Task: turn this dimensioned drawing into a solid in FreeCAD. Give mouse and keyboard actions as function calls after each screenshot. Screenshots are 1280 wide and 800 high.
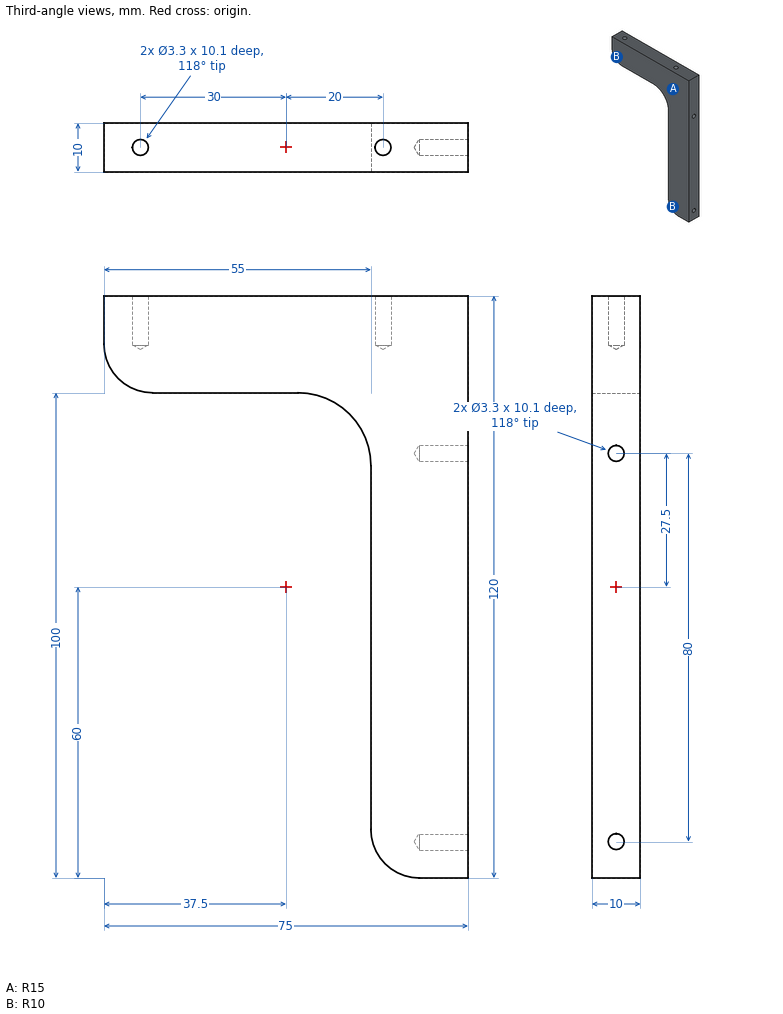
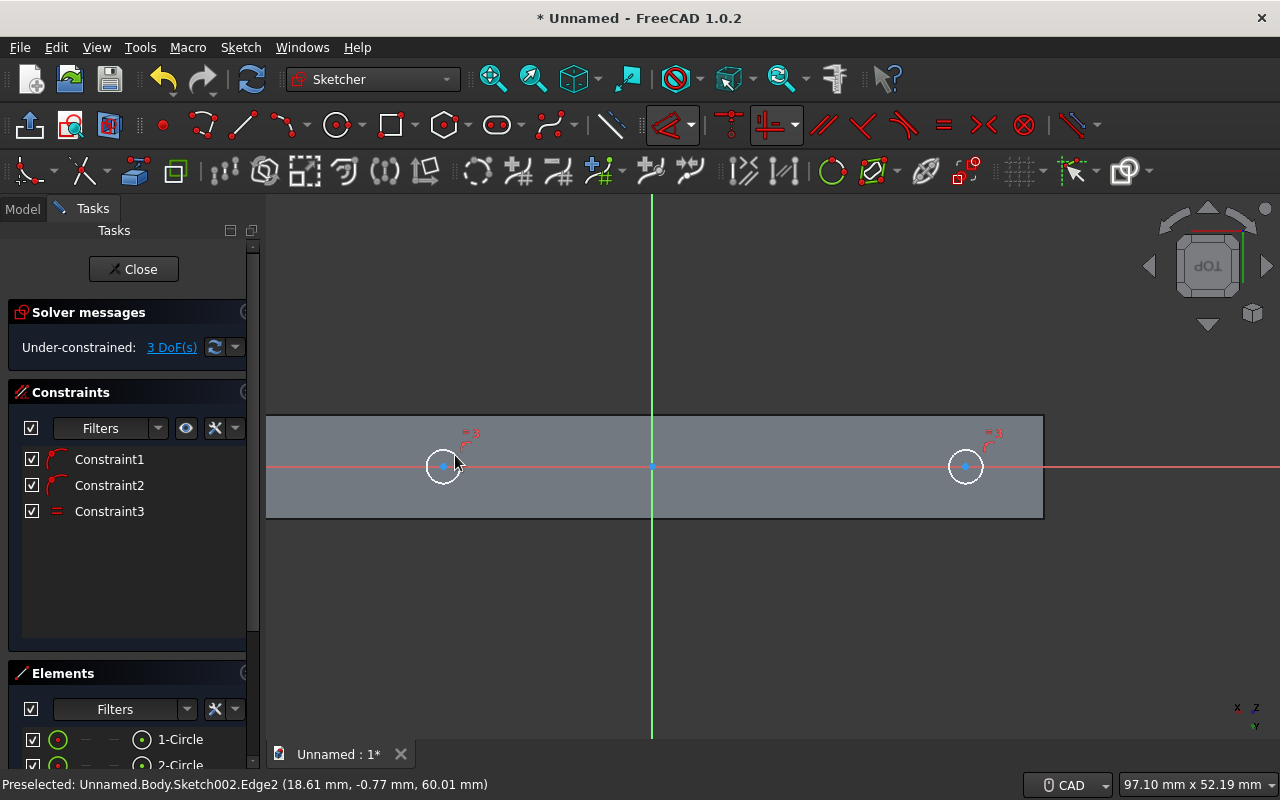
key(d)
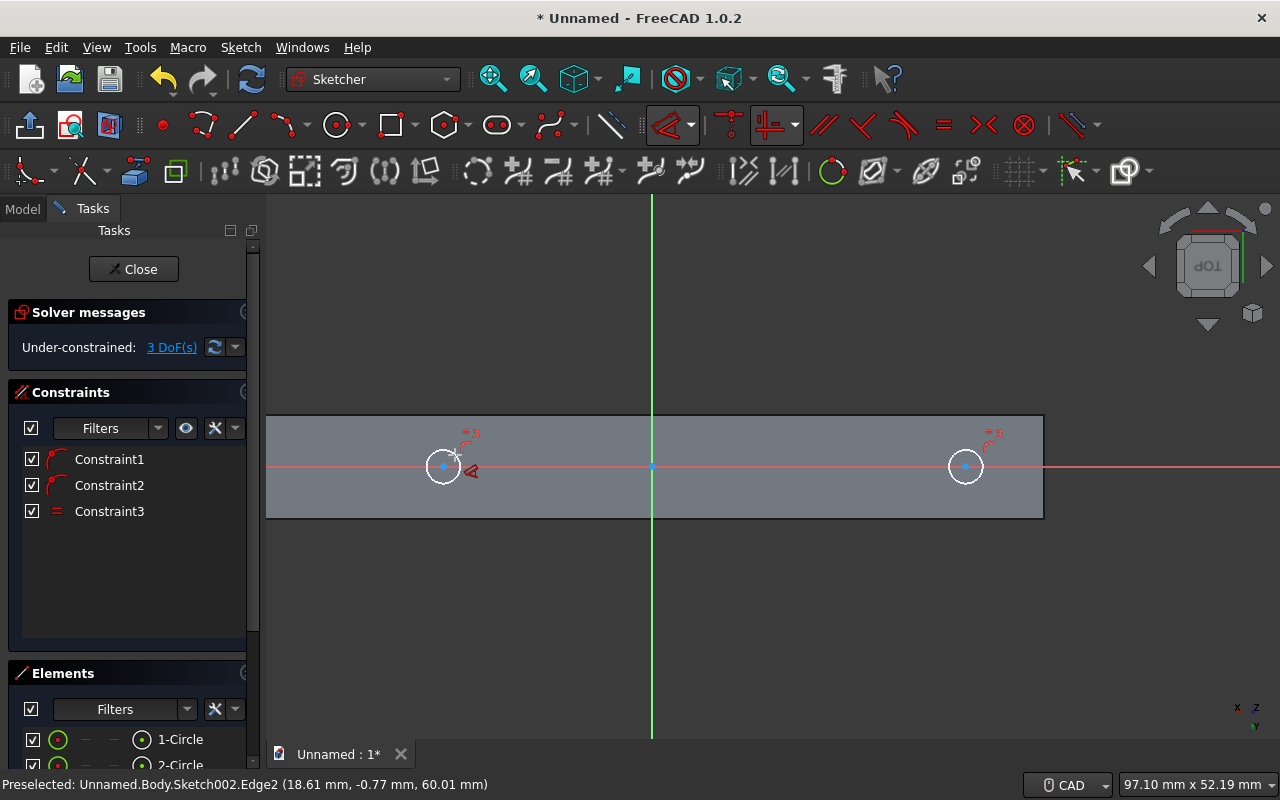
click(978, 455)
click(1001, 433)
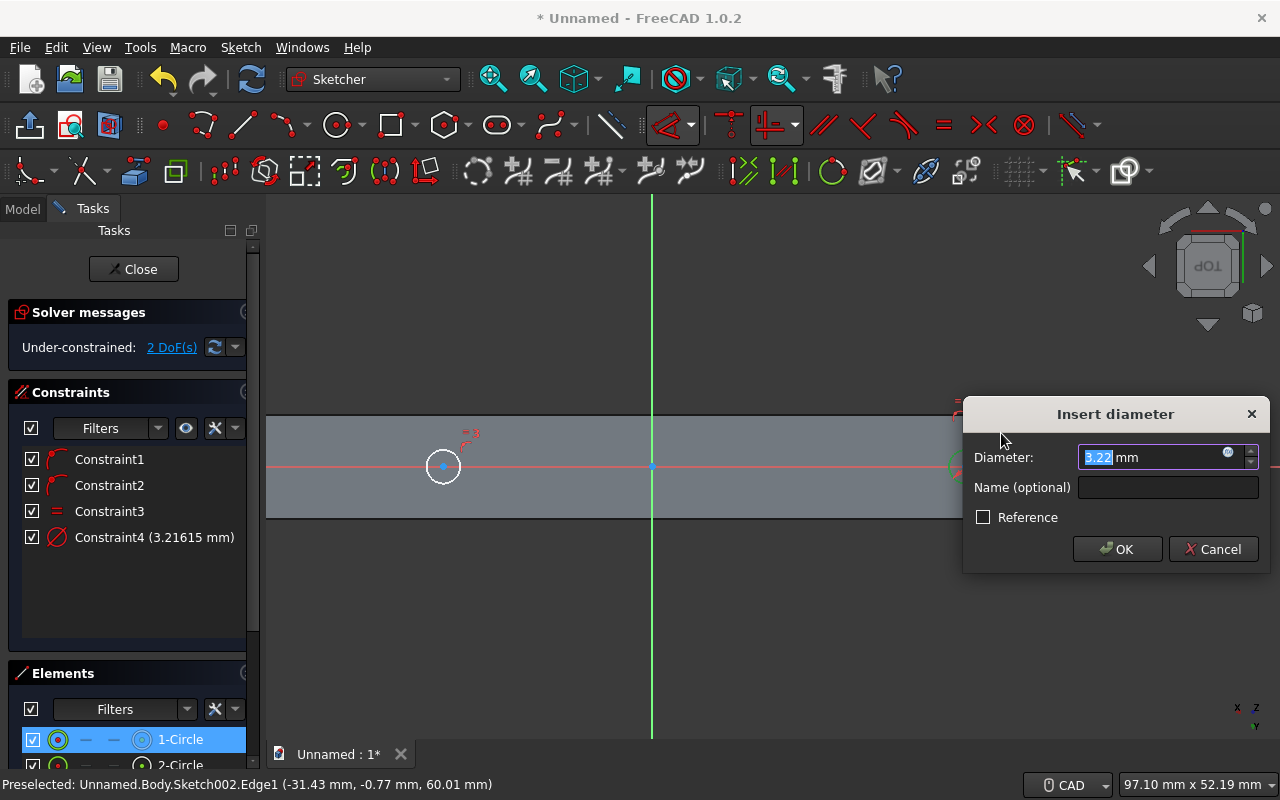
text(3.3)
key(Return)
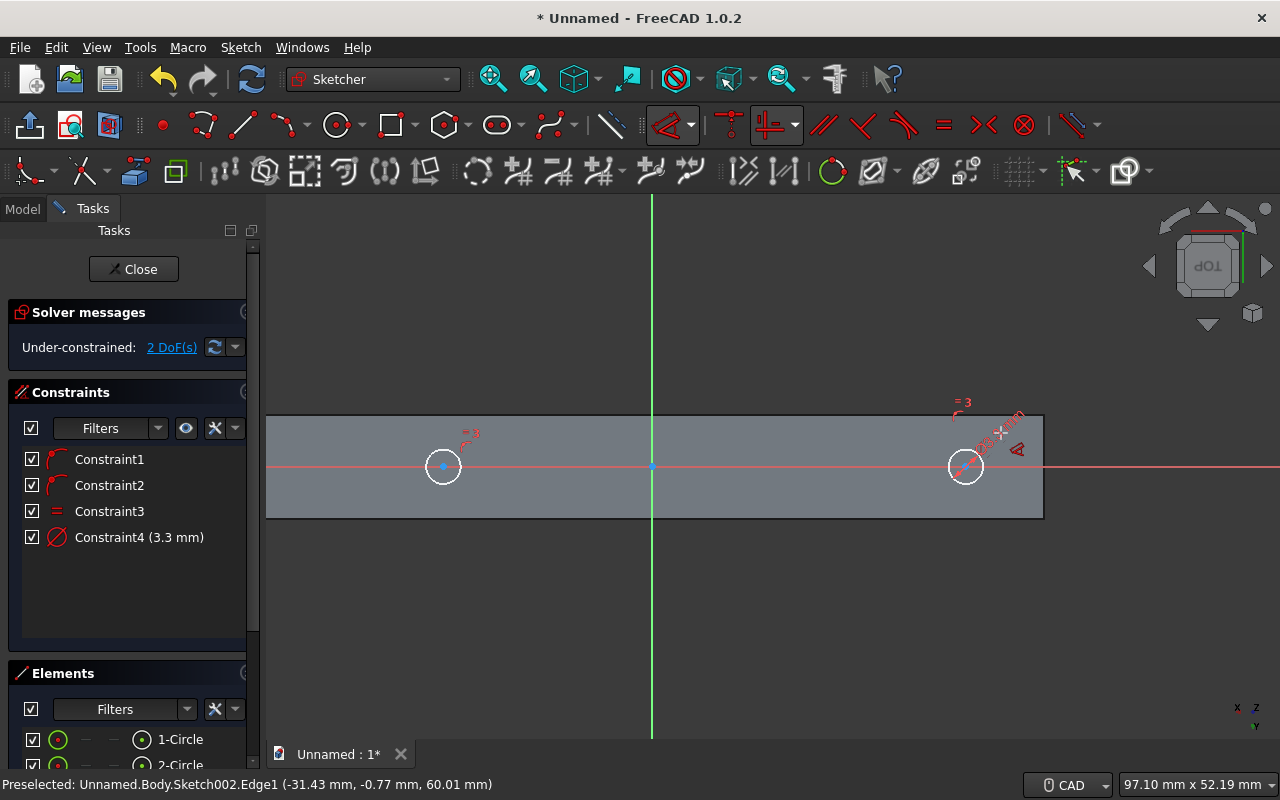
click(966, 467)
click(809, 501)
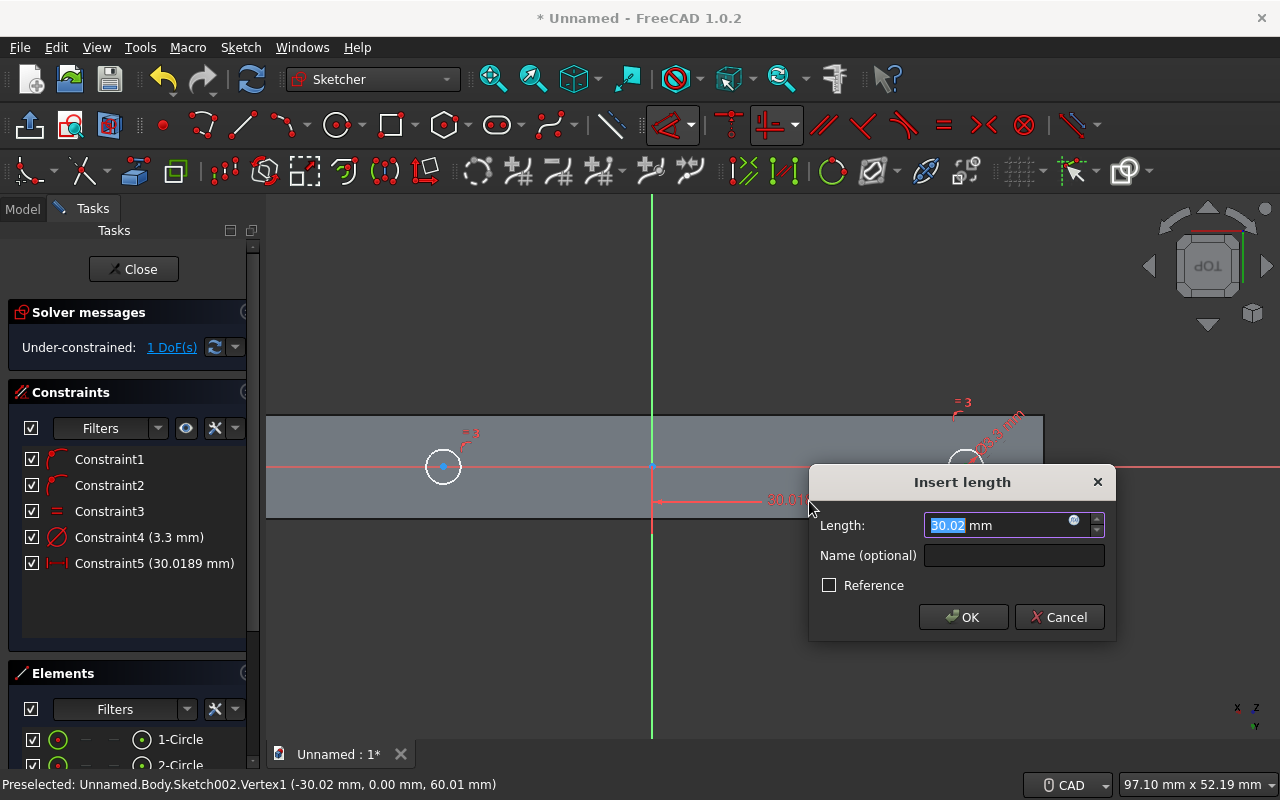
text(30)
key(Return)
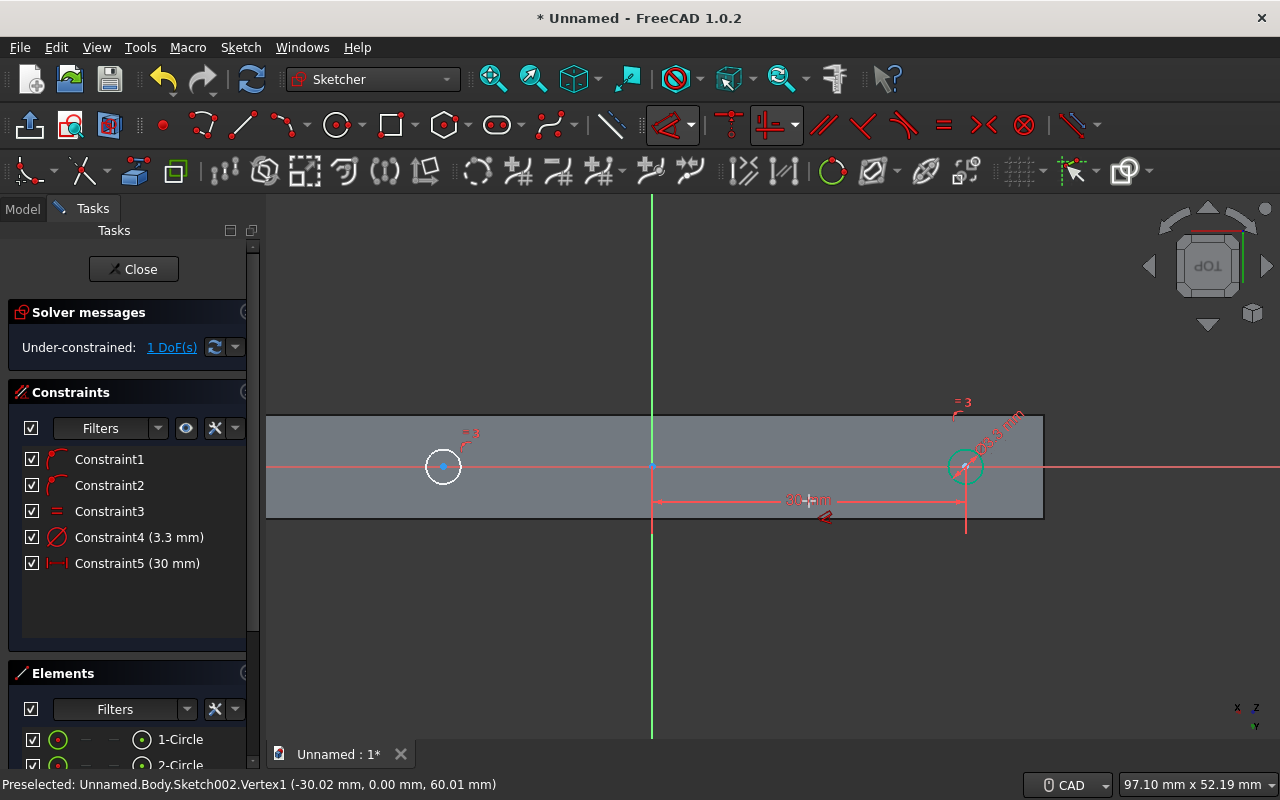
click(443, 467)
click(548, 501)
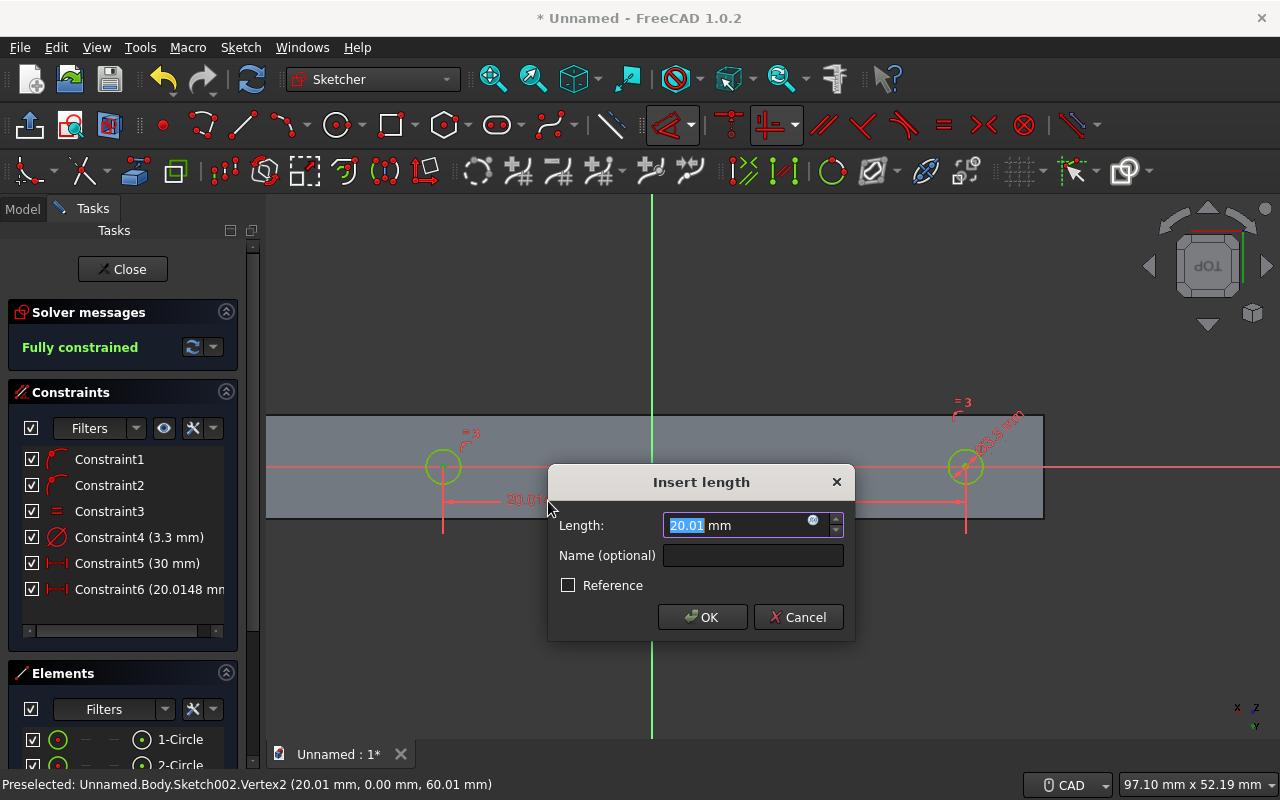
text(20)
key(Return)
key(Escape)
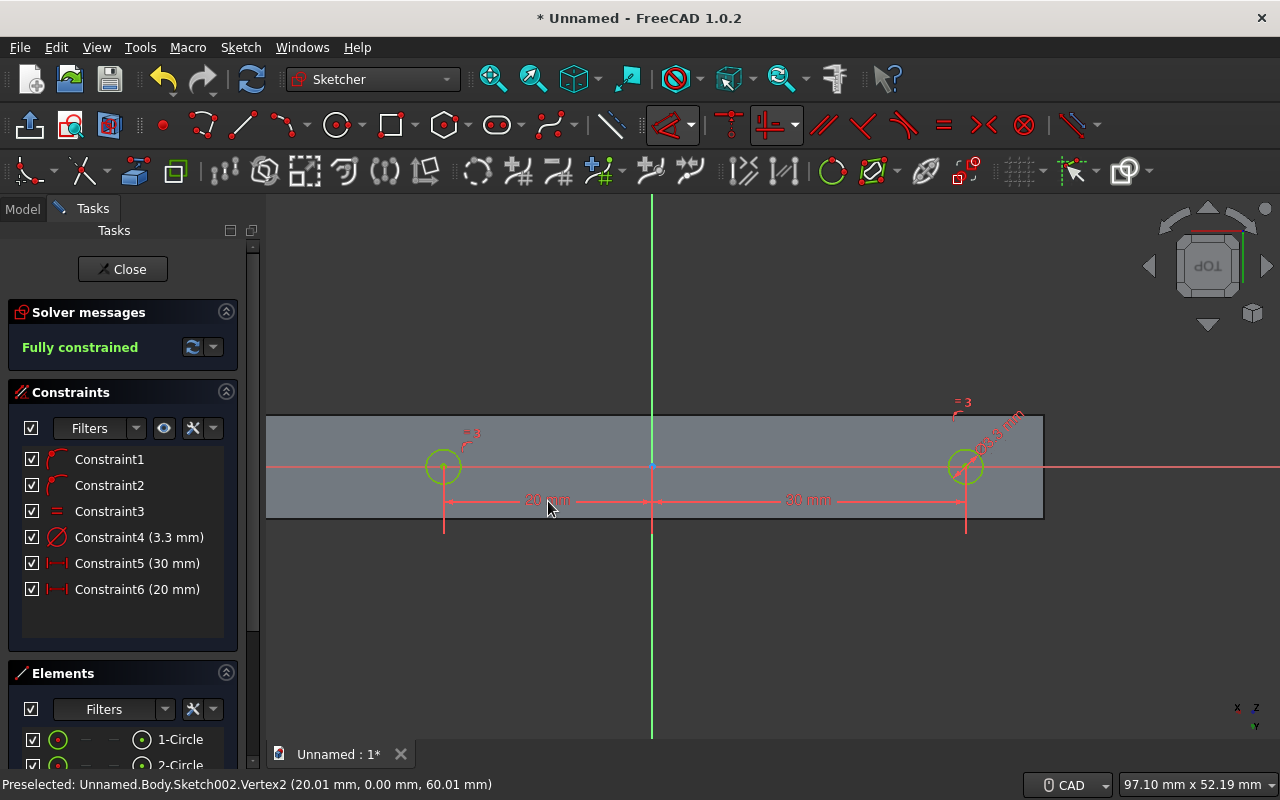
click(123, 269)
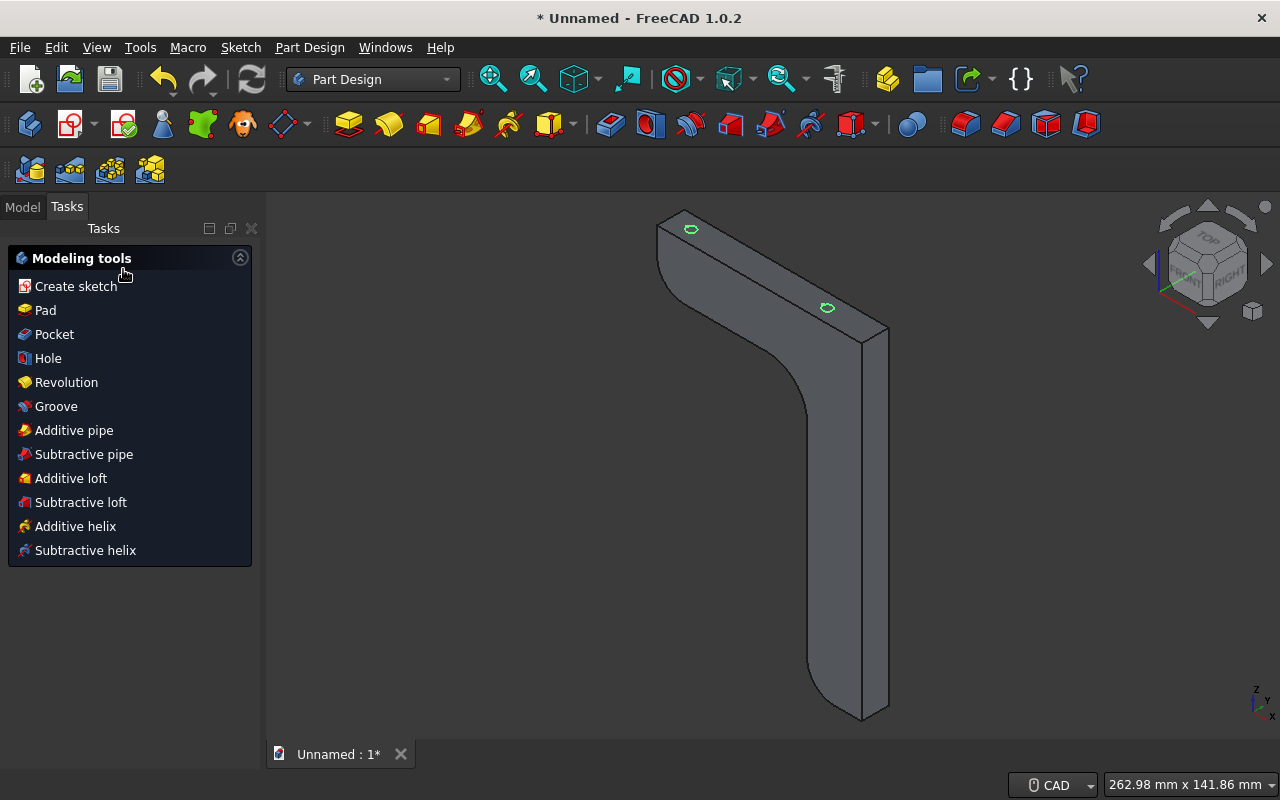
click(652, 124)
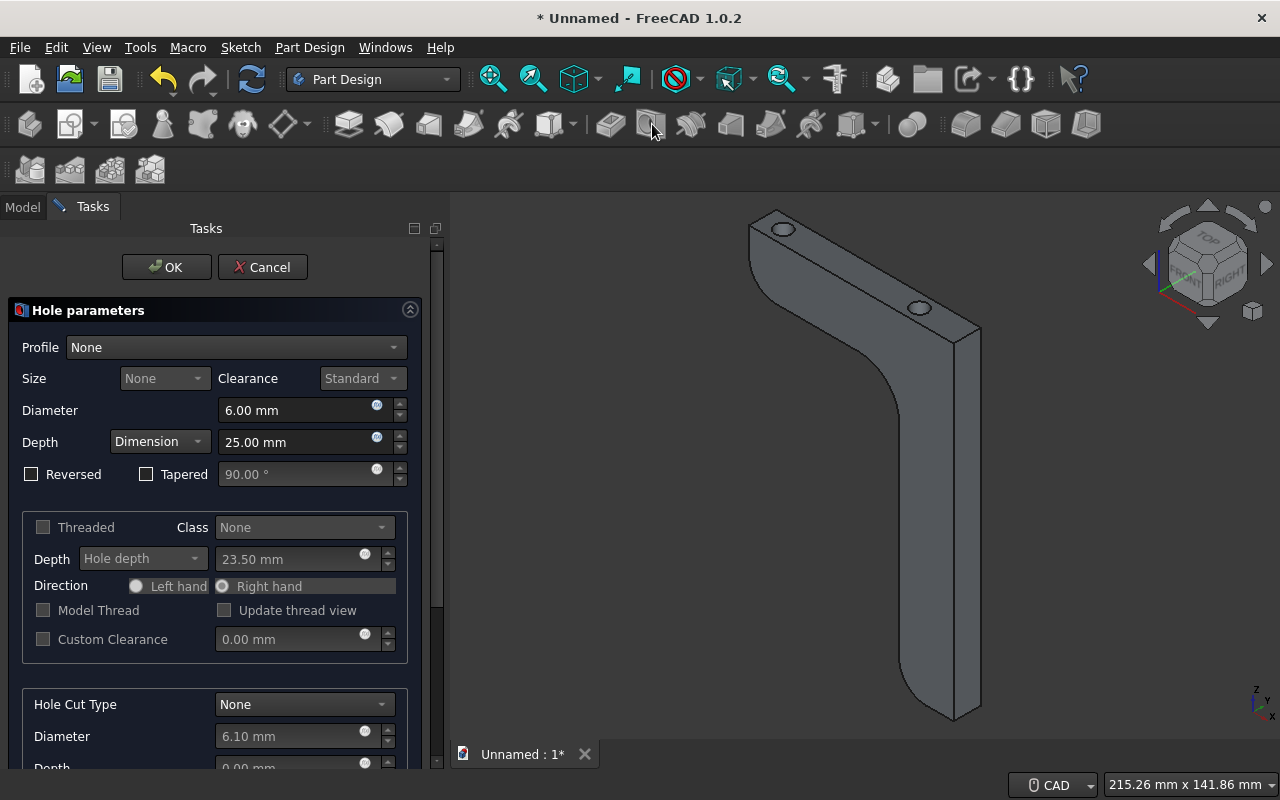
triple_click(305, 410)